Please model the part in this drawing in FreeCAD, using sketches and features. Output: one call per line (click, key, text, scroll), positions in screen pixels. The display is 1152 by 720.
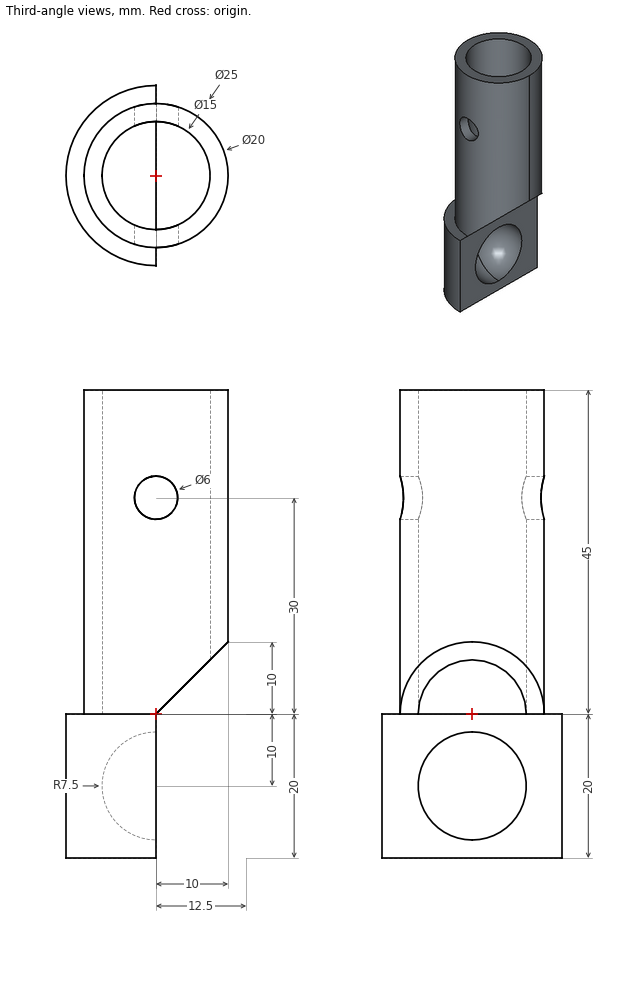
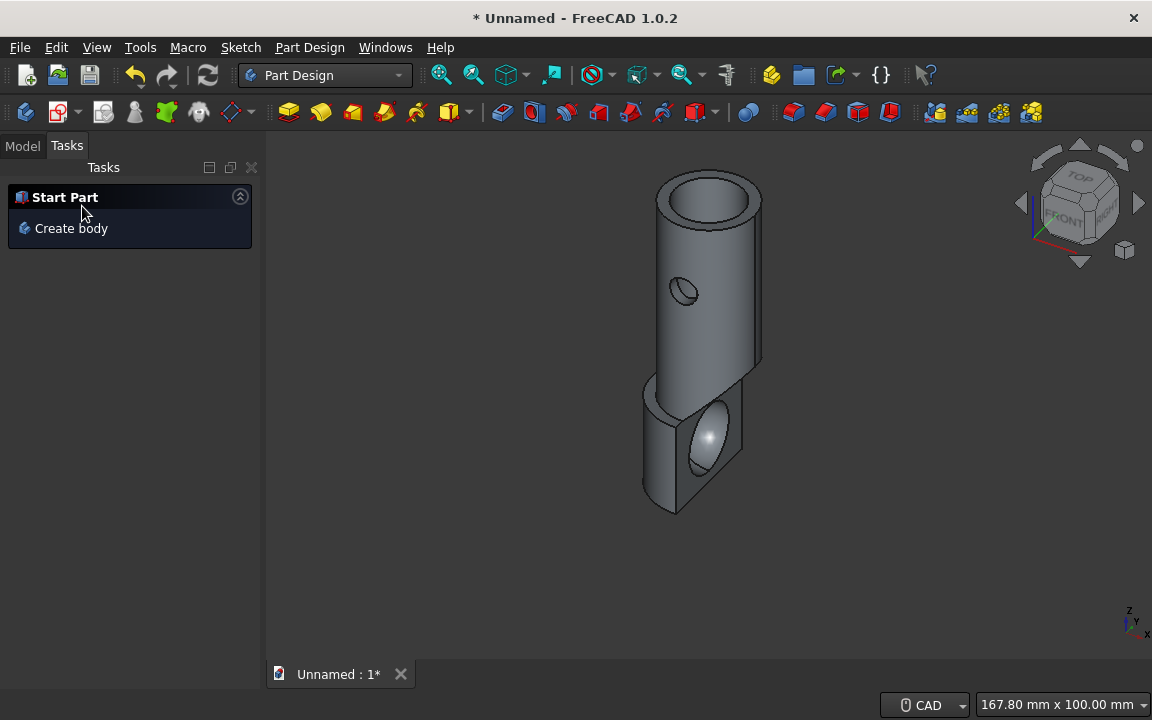
key(0)